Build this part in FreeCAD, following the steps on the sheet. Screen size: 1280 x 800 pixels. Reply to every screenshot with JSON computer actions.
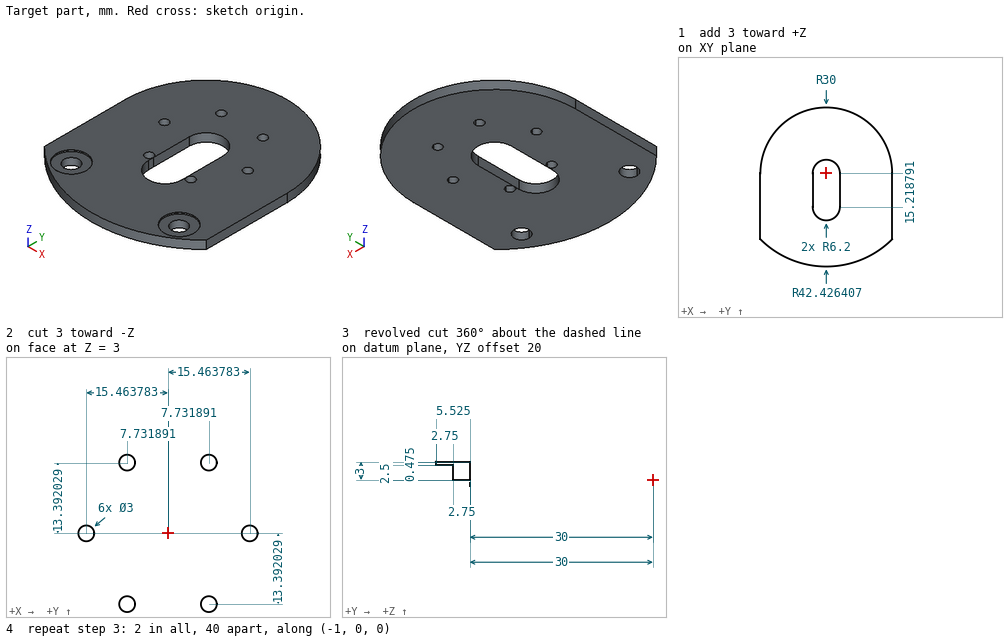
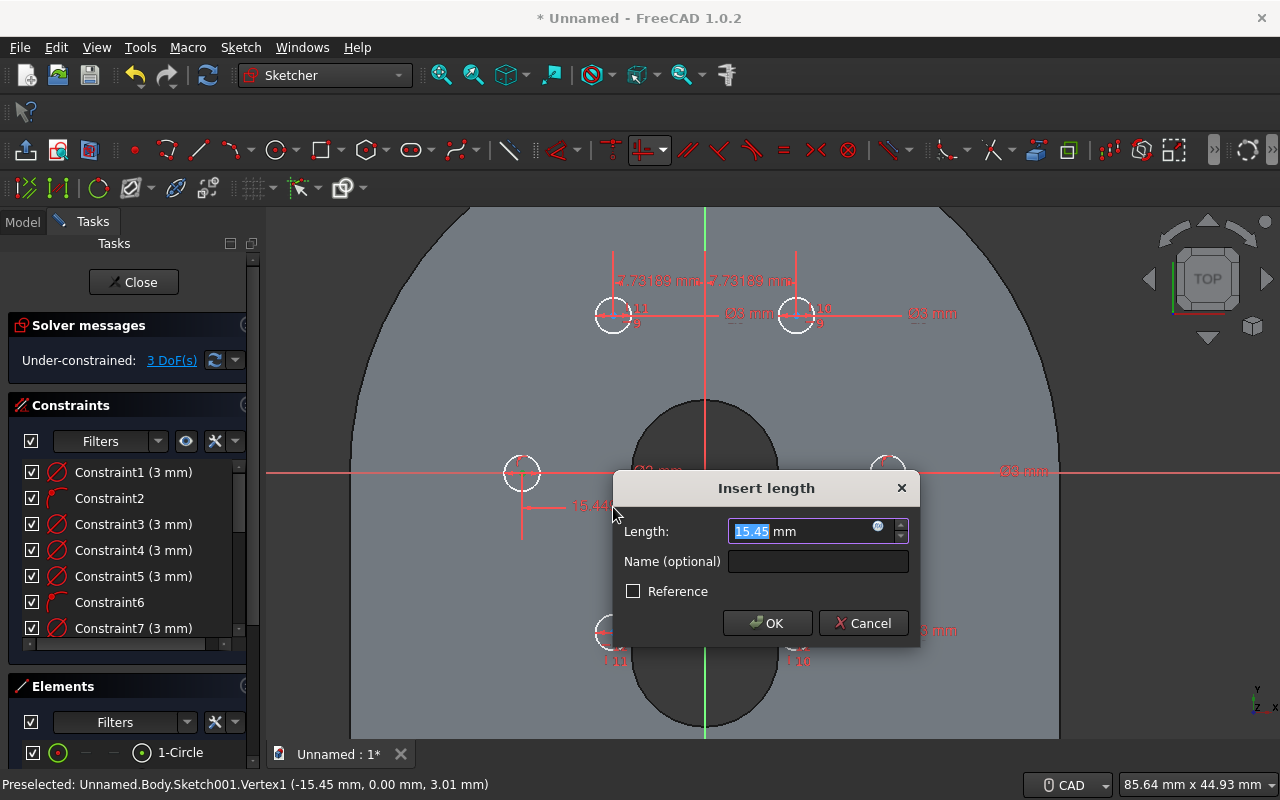
{"action": "type", "text": "15.463783"}
{"action": "key", "text": "Return"}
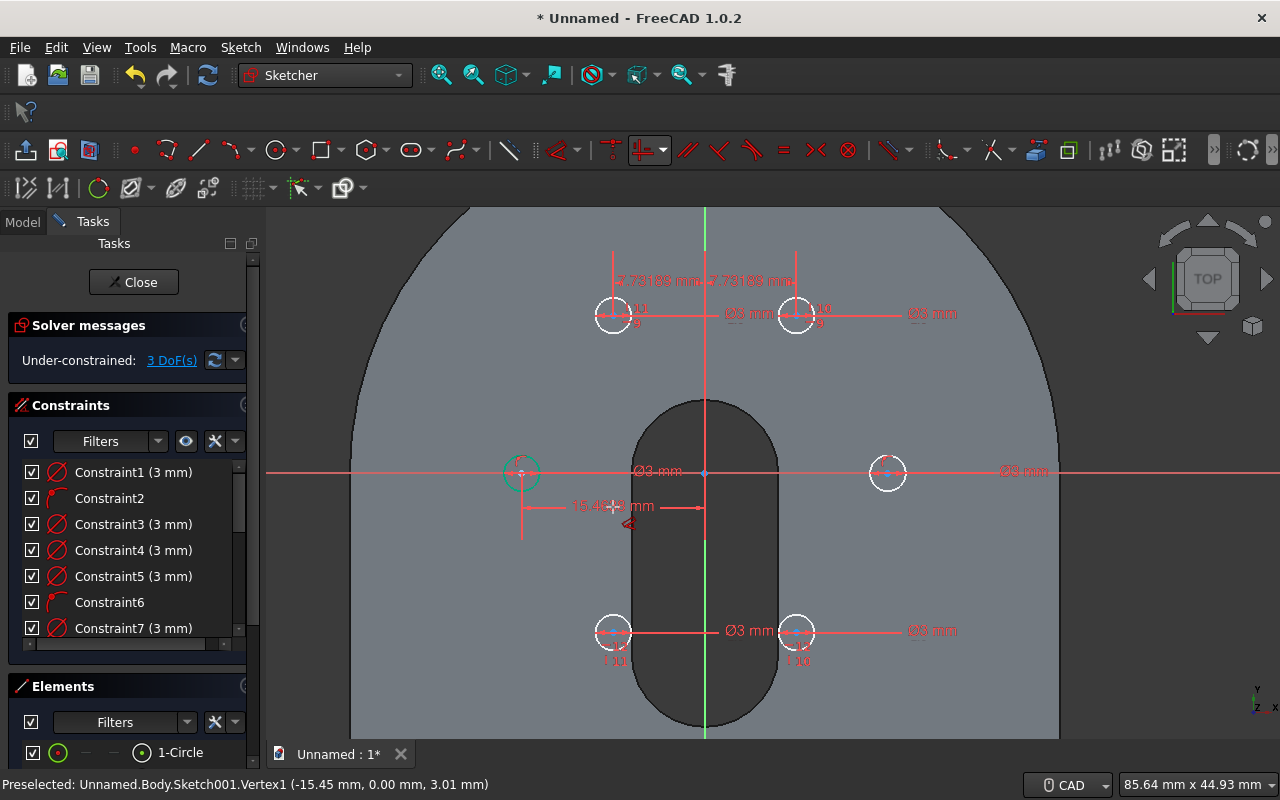
{"action": "left_click", "coordinate": [613, 316]}
{"action": "left_click", "coordinate": [579, 394]}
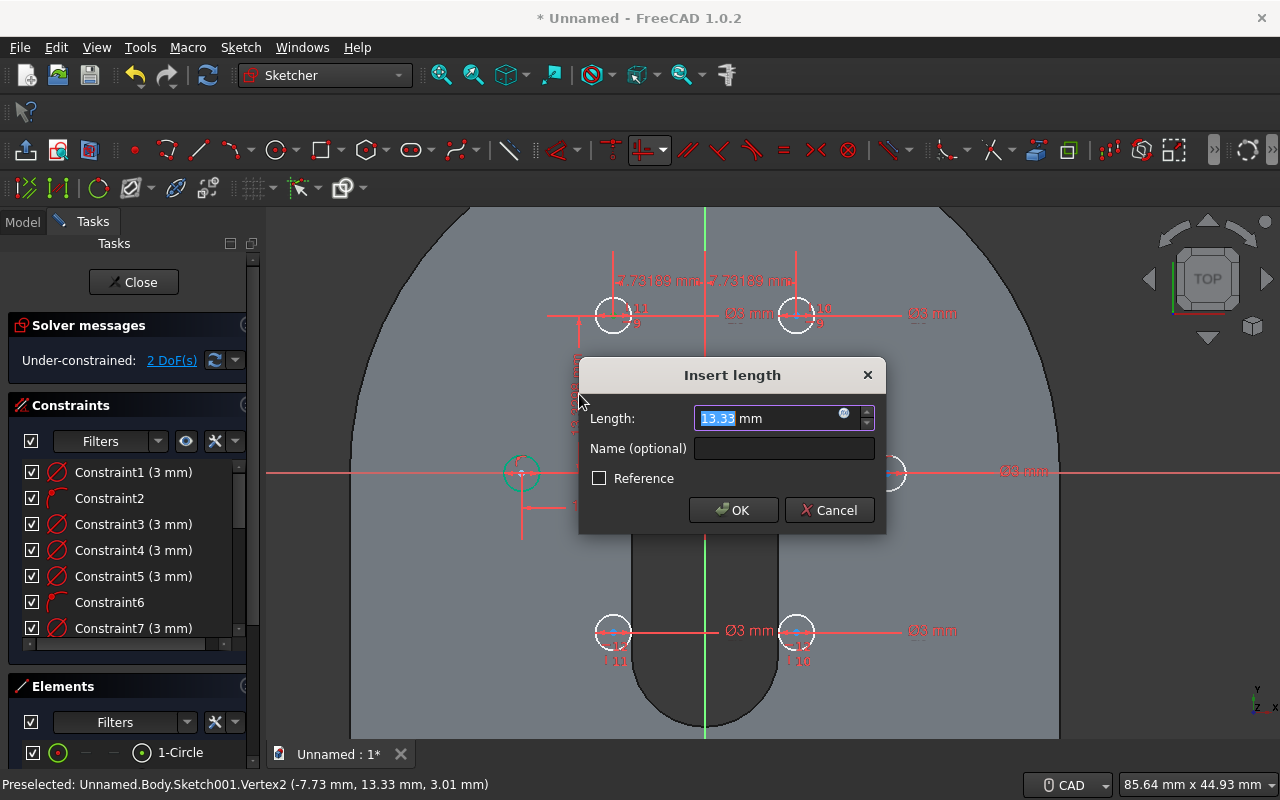
{"action": "type", "text": "13.392029"}
{"action": "key", "text": "Return"}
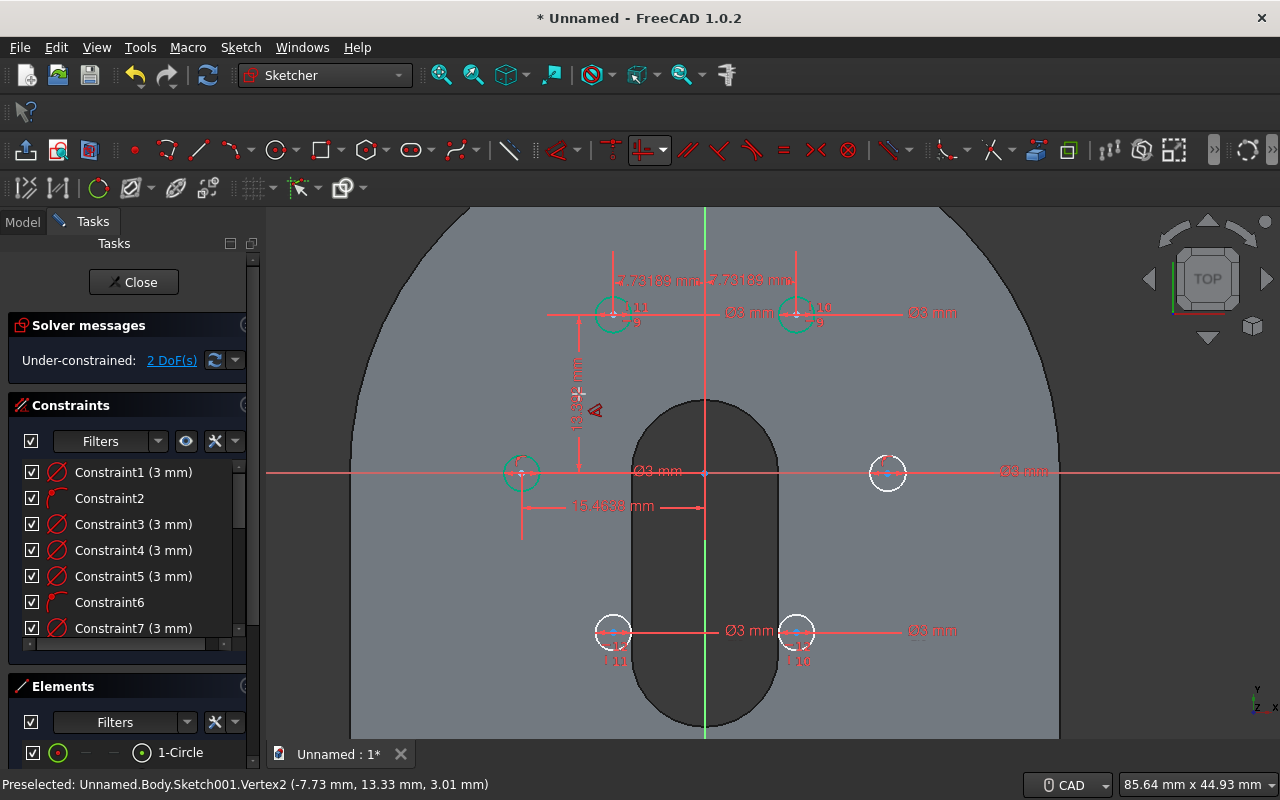
{"action": "left_click", "coordinate": [888, 473]}
{"action": "left_click", "coordinate": [796, 507]}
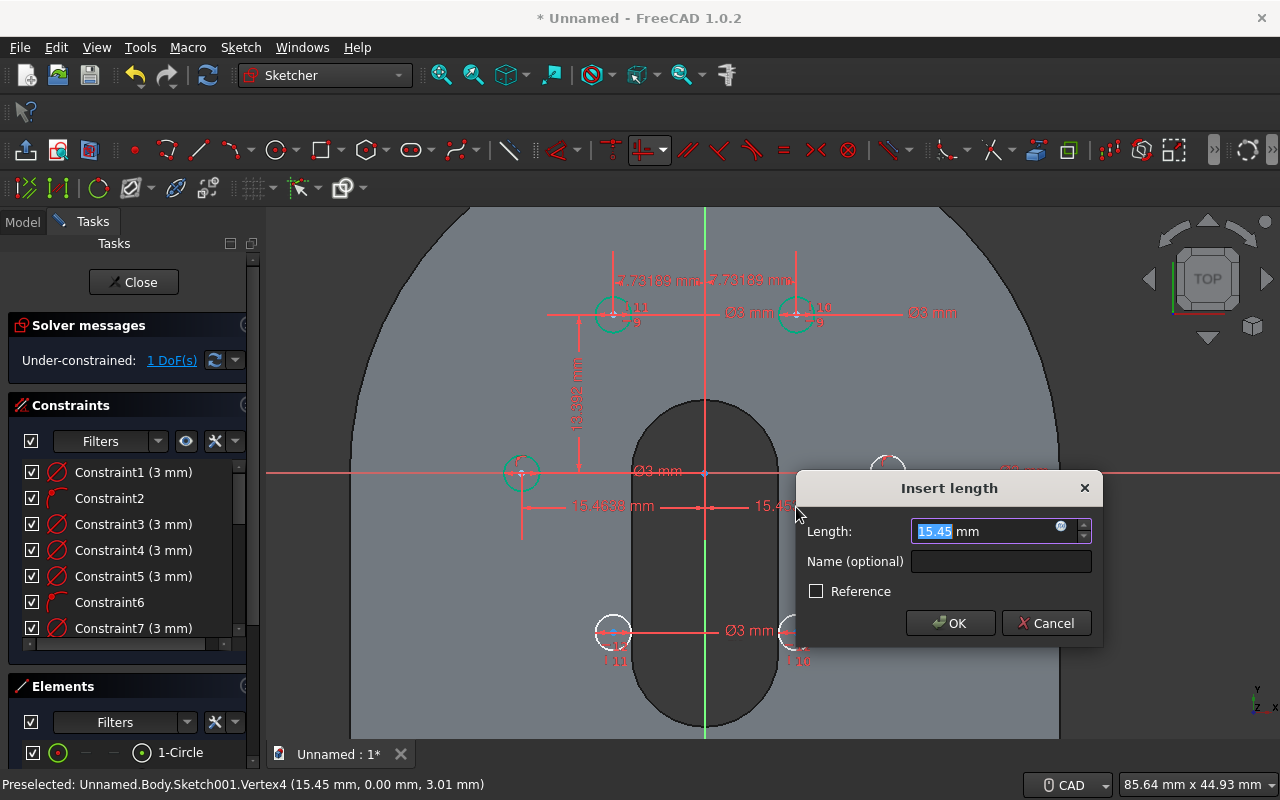
{"action": "type", "text": "15.463783"}
{"action": "key", "text": "Return"}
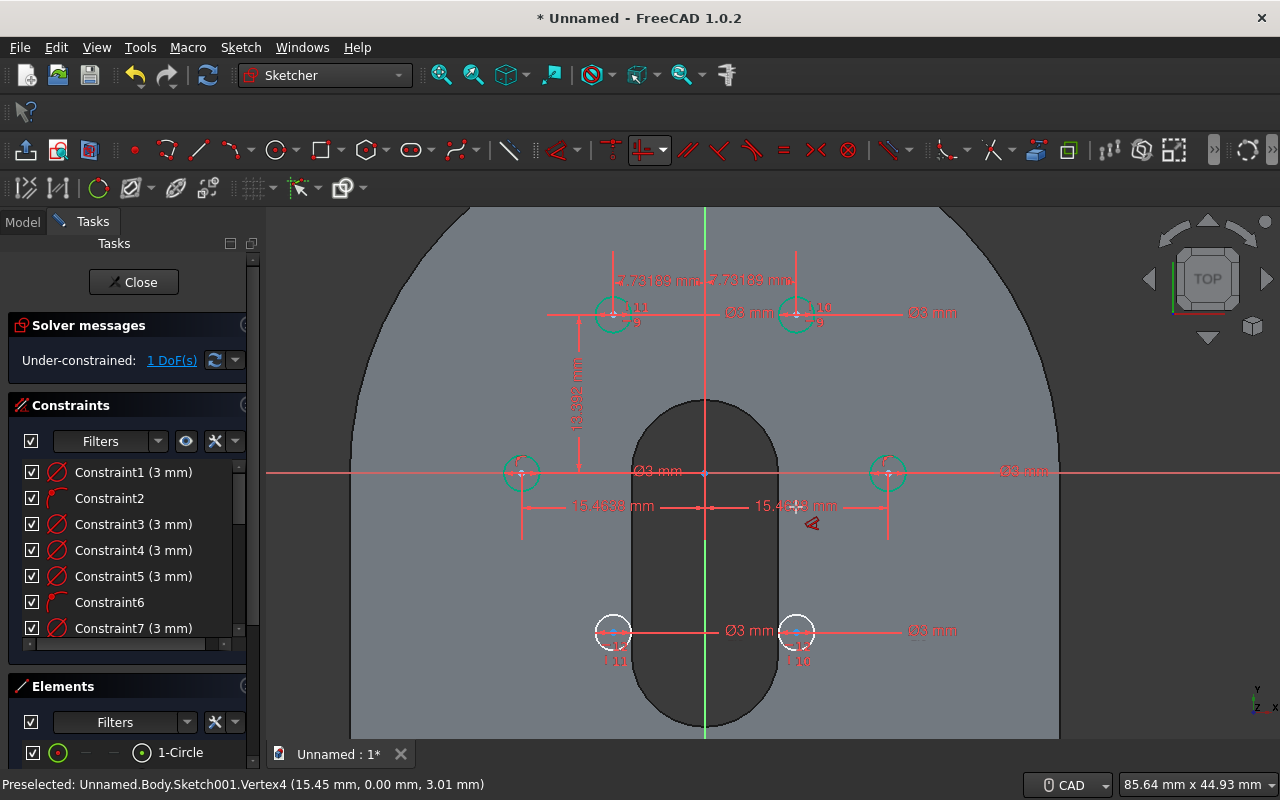
{"action": "left_click", "coordinate": [796, 633]}
{"action": "left_click", "coordinate": [830, 553]}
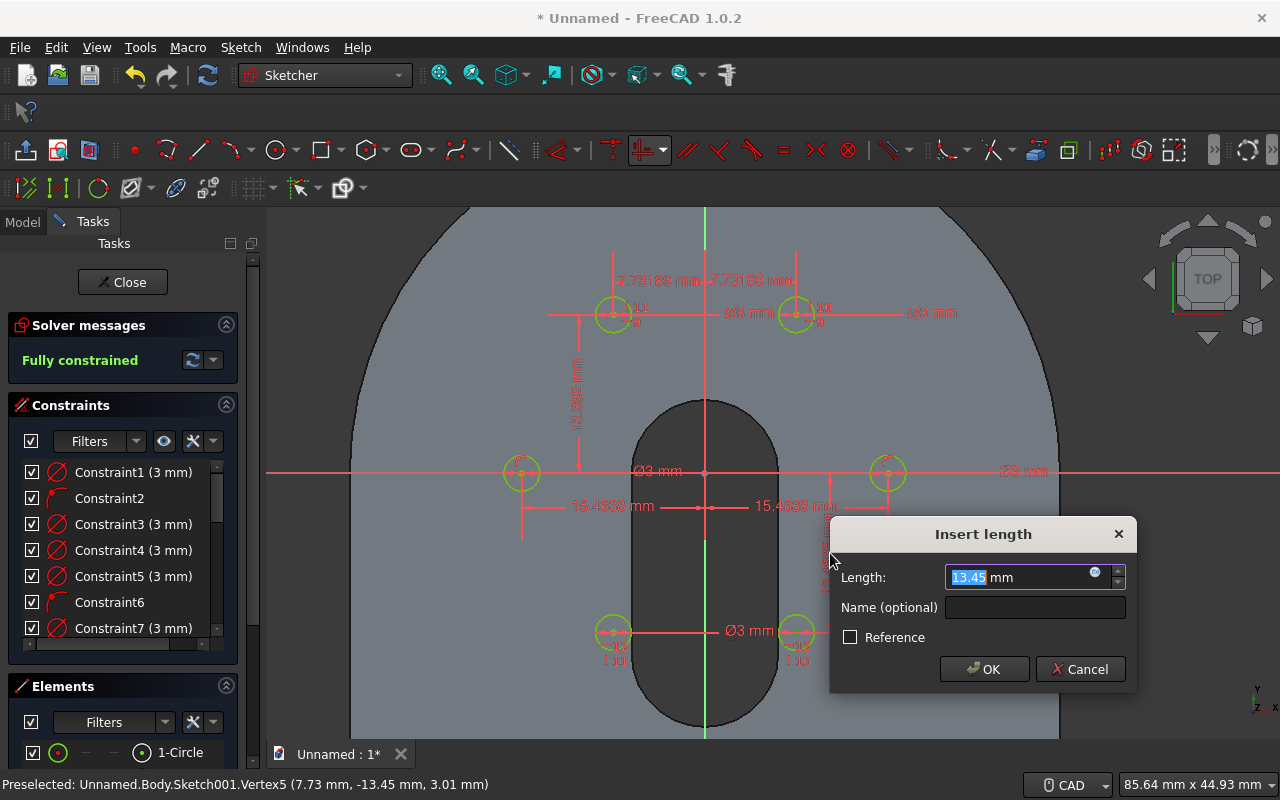
{"action": "type", "text": "13.392029"}
{"action": "key", "text": "Return"}
{"action": "key", "text": "Escape"}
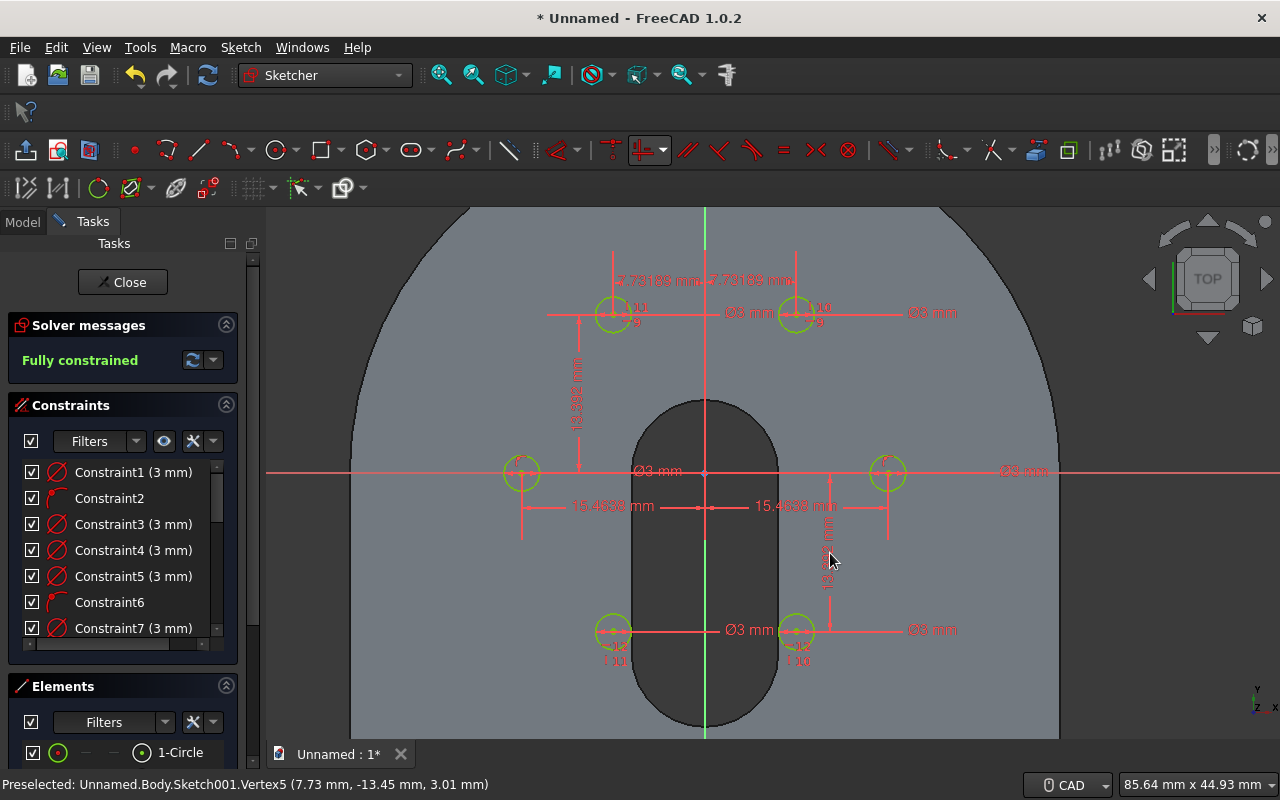
{"action": "left_click", "coordinate": [123, 282]}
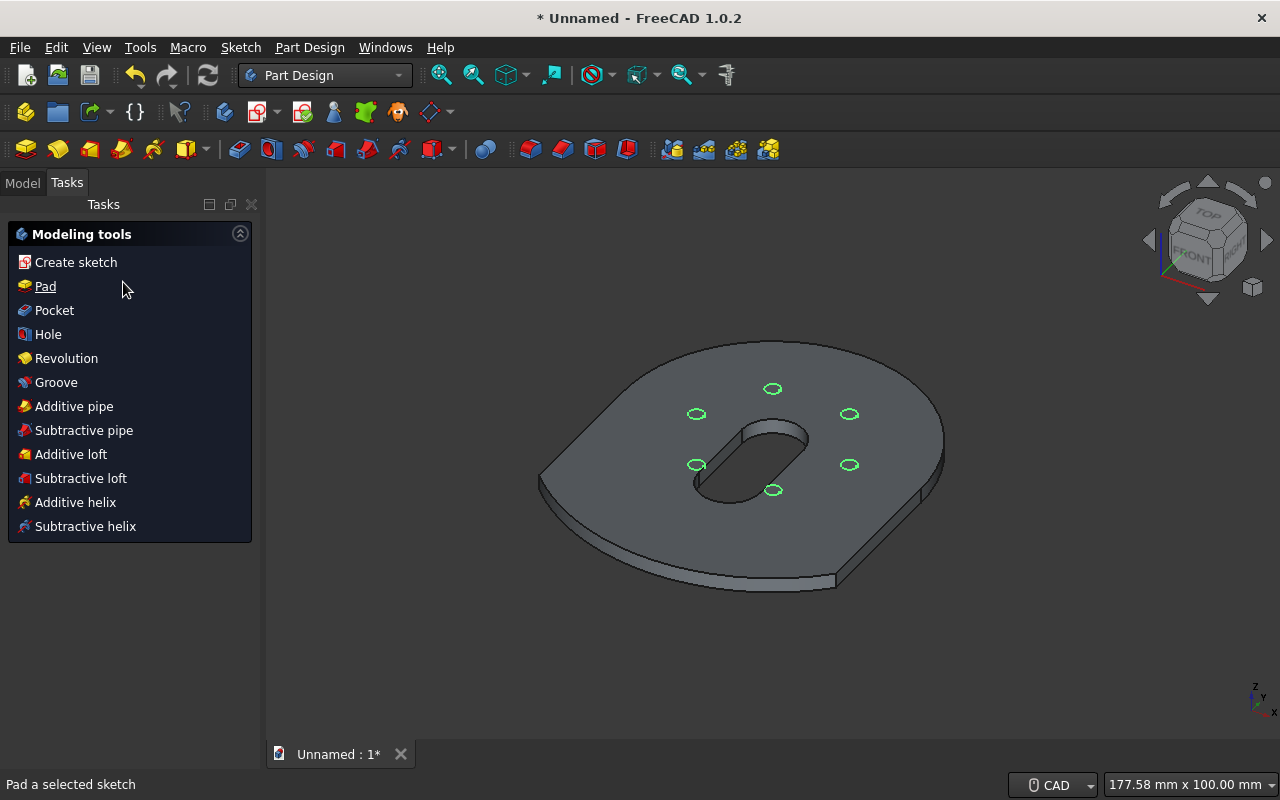
{"action": "left_click", "coordinate": [240, 150]}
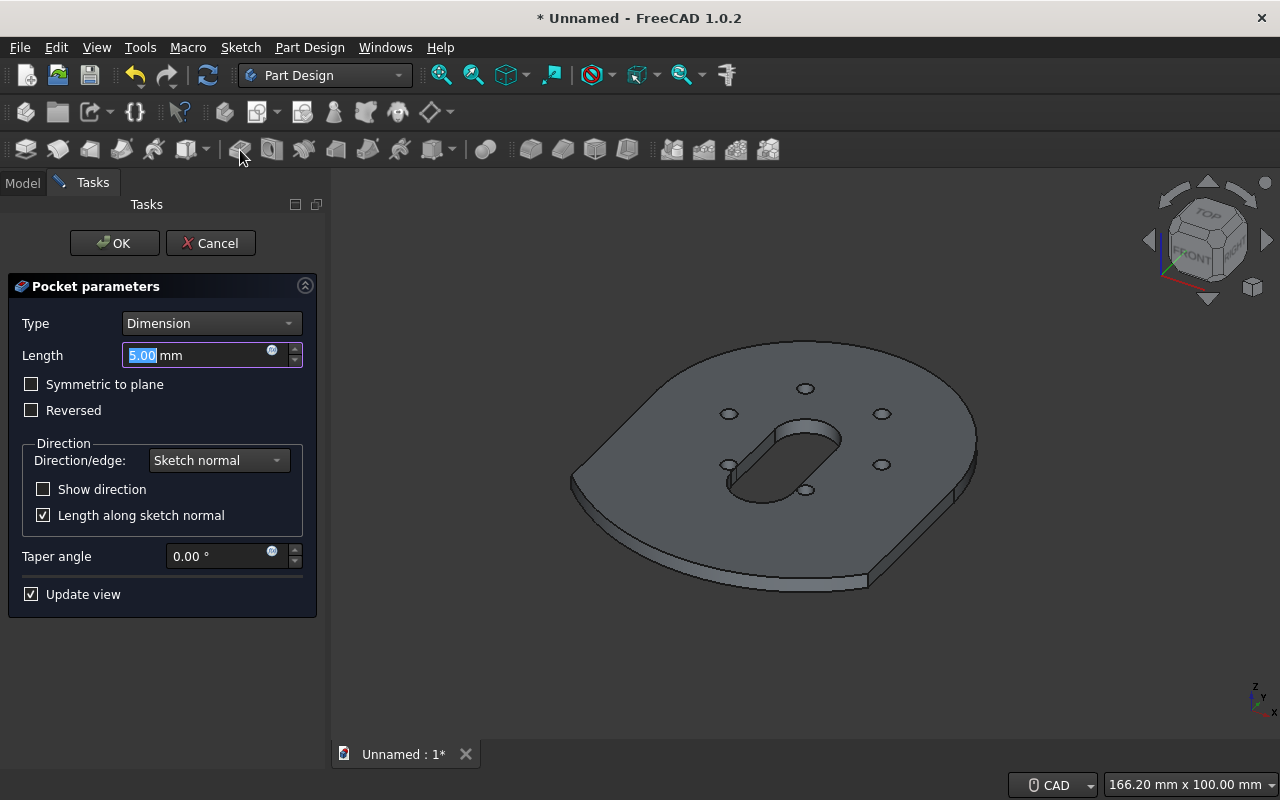
{"action": "type", "text": "3"}
{"action": "key", "text": "Tab"}